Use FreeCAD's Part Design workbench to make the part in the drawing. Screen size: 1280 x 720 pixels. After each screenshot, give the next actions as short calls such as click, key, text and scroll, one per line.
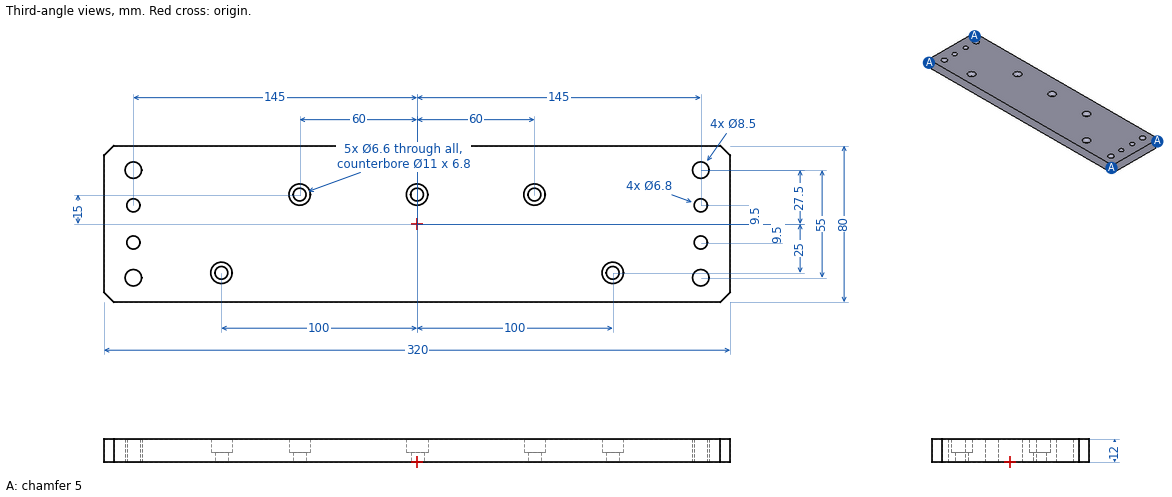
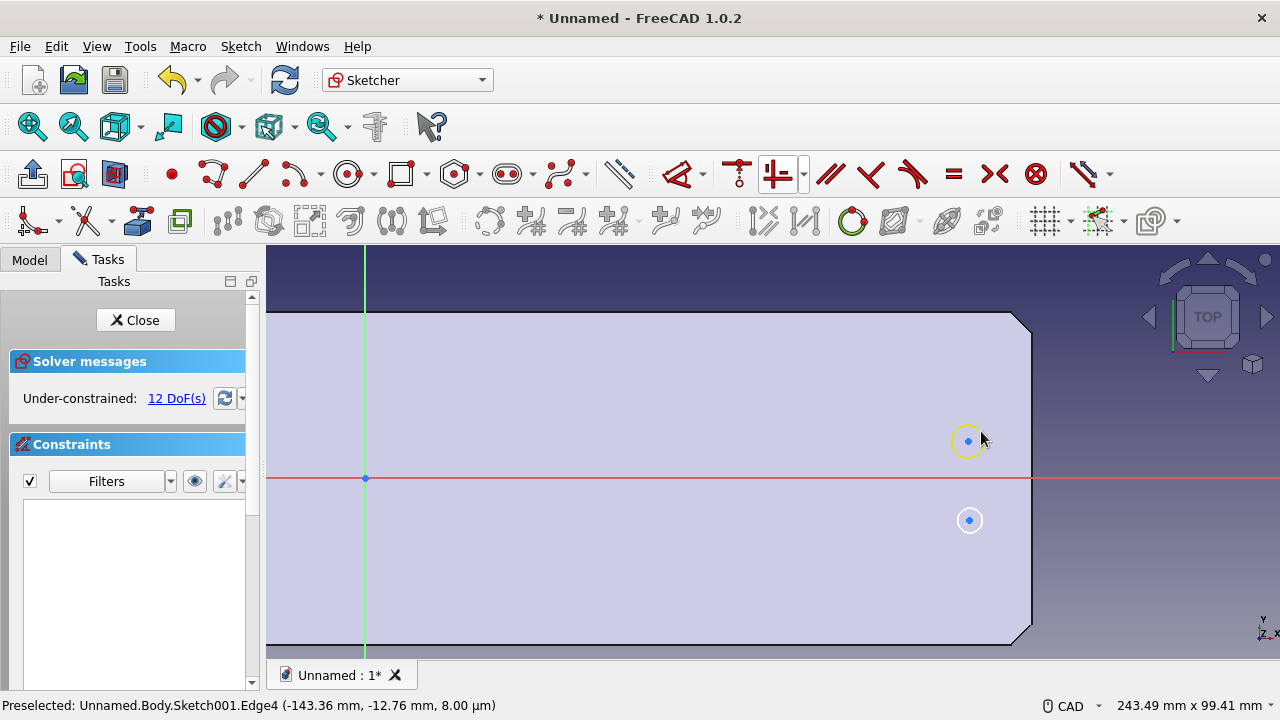
click(980, 430)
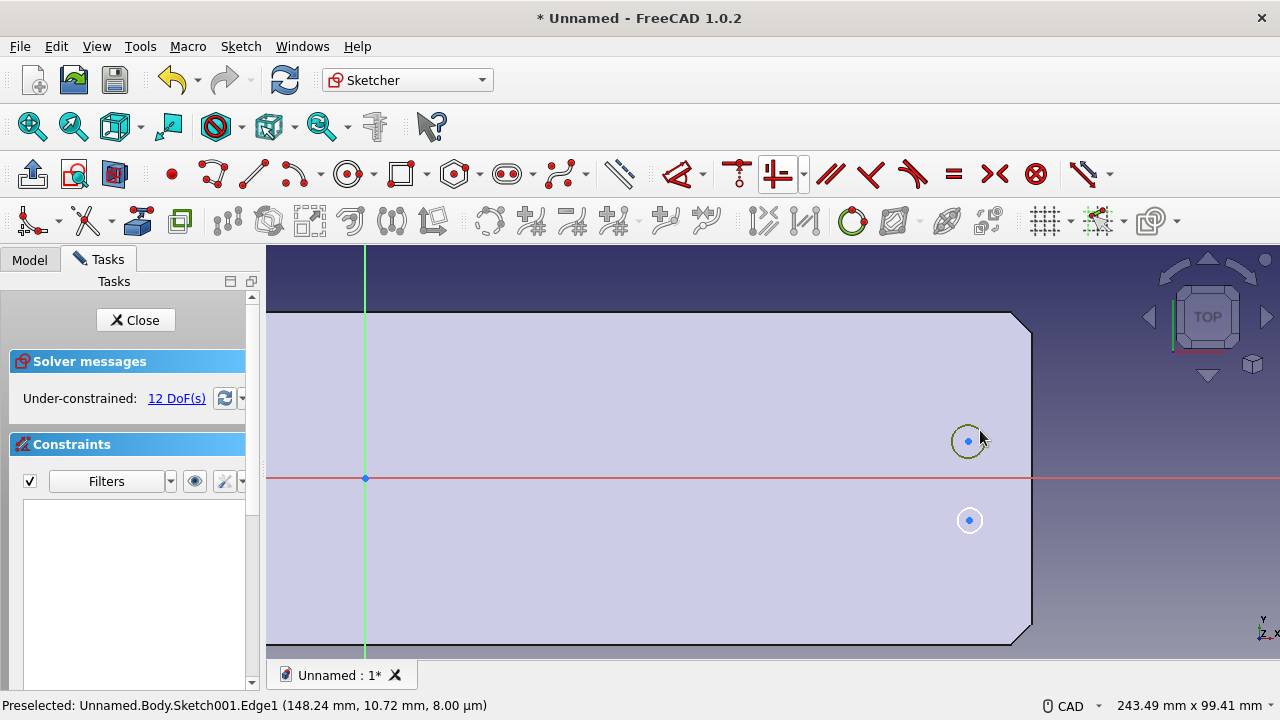
click(979, 512)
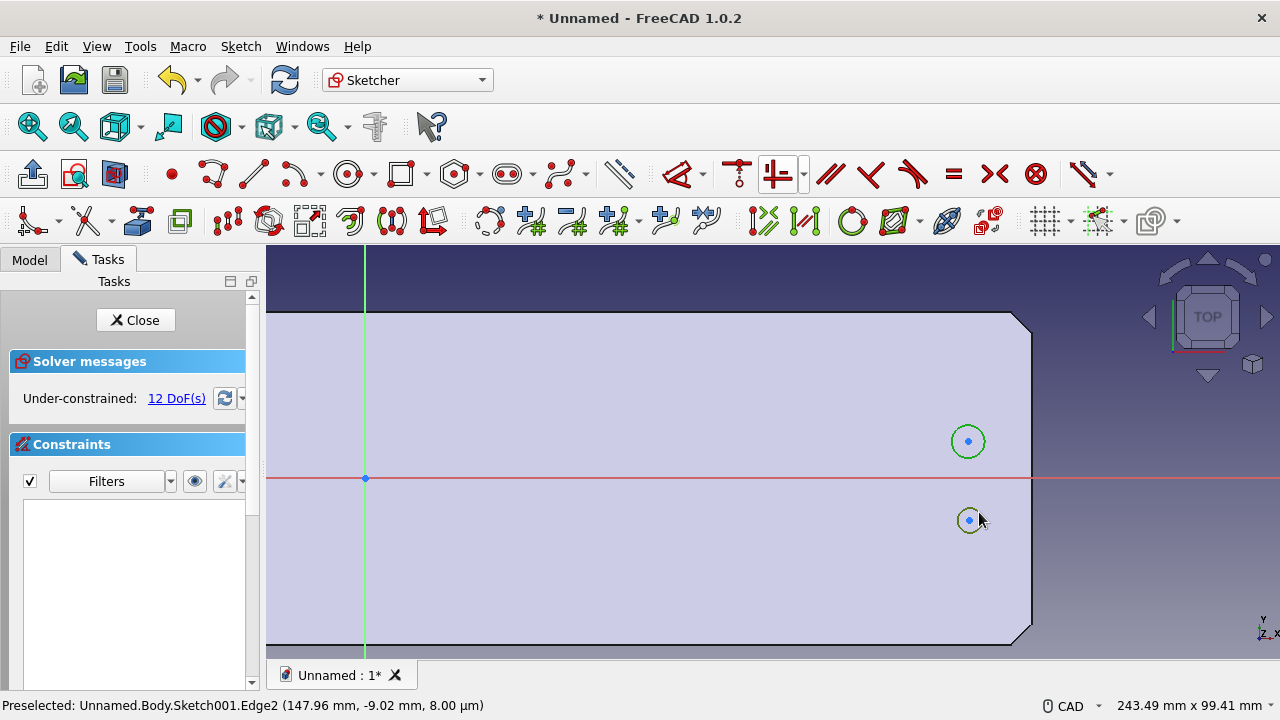
scroll(981, 430, down, 4)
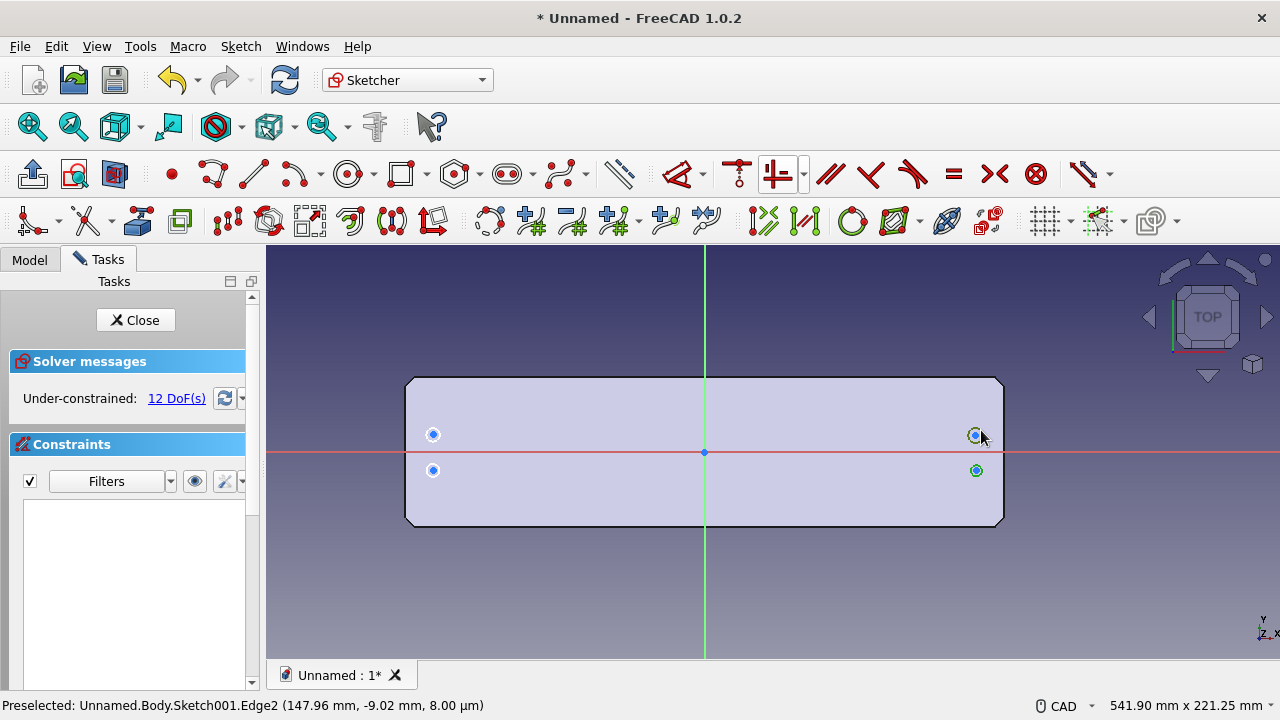
scroll(438, 430, up, 4)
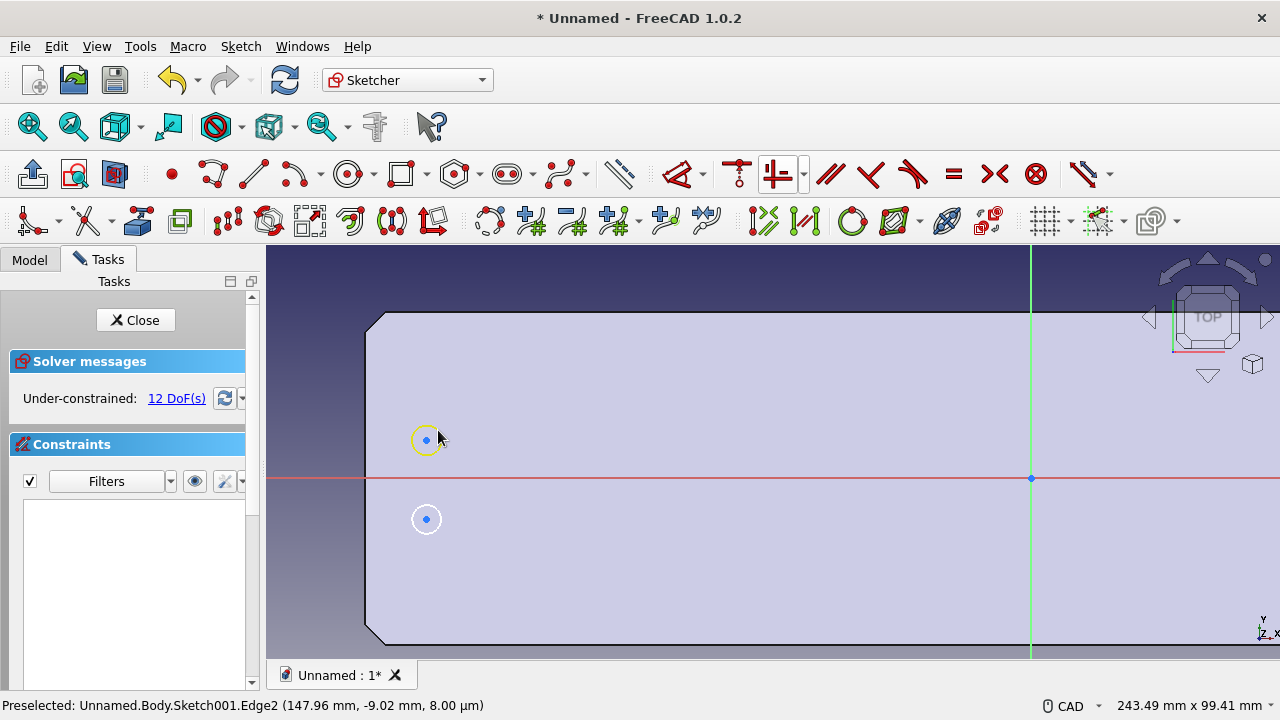
click(437, 430)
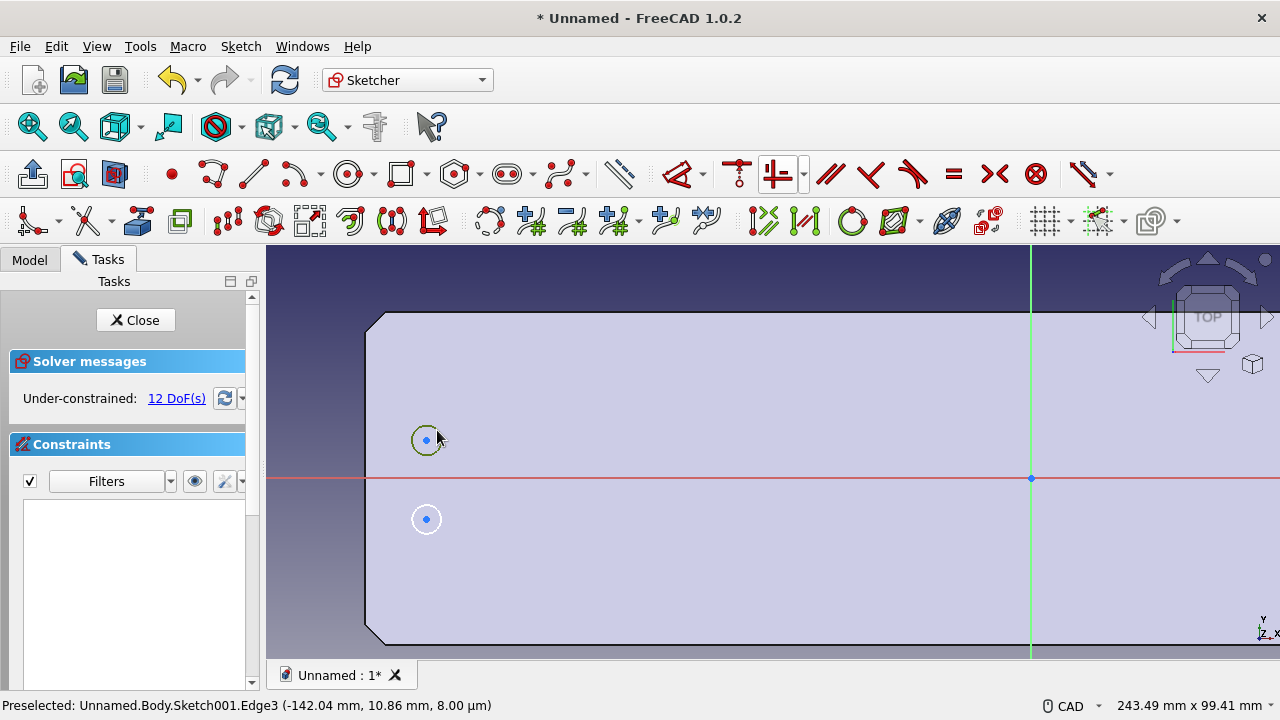
click(437, 509)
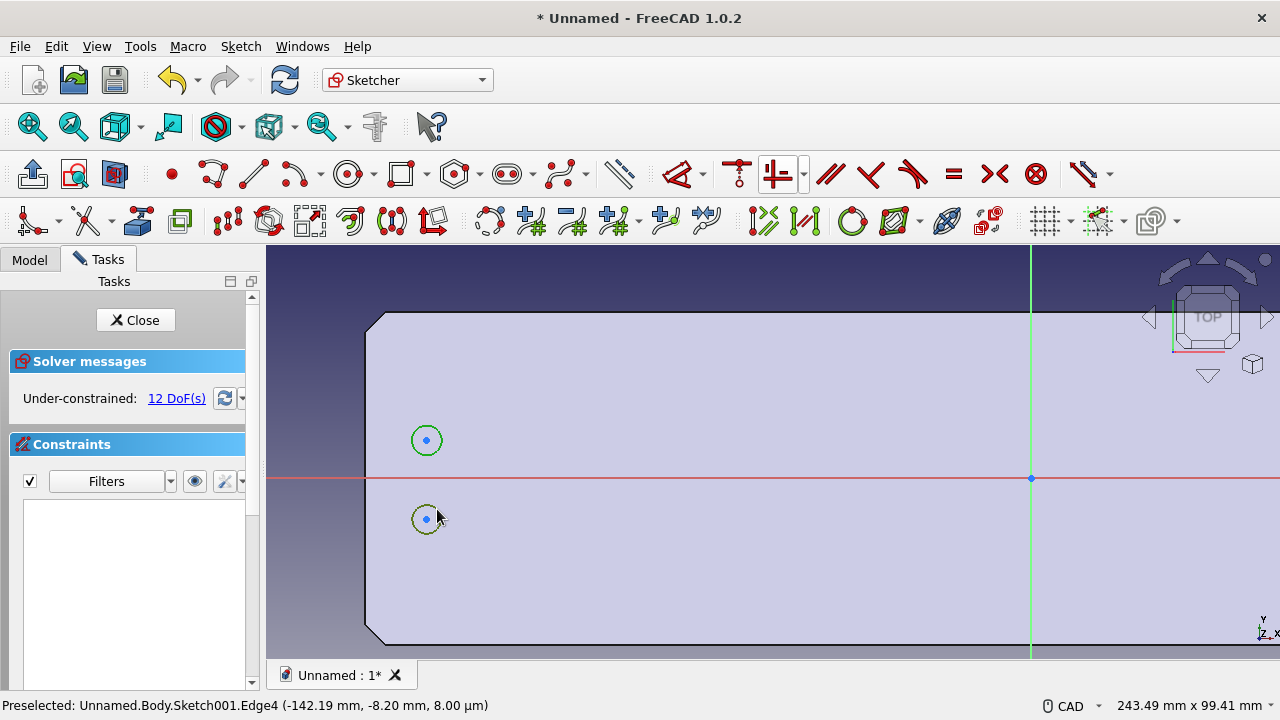
click(954, 174)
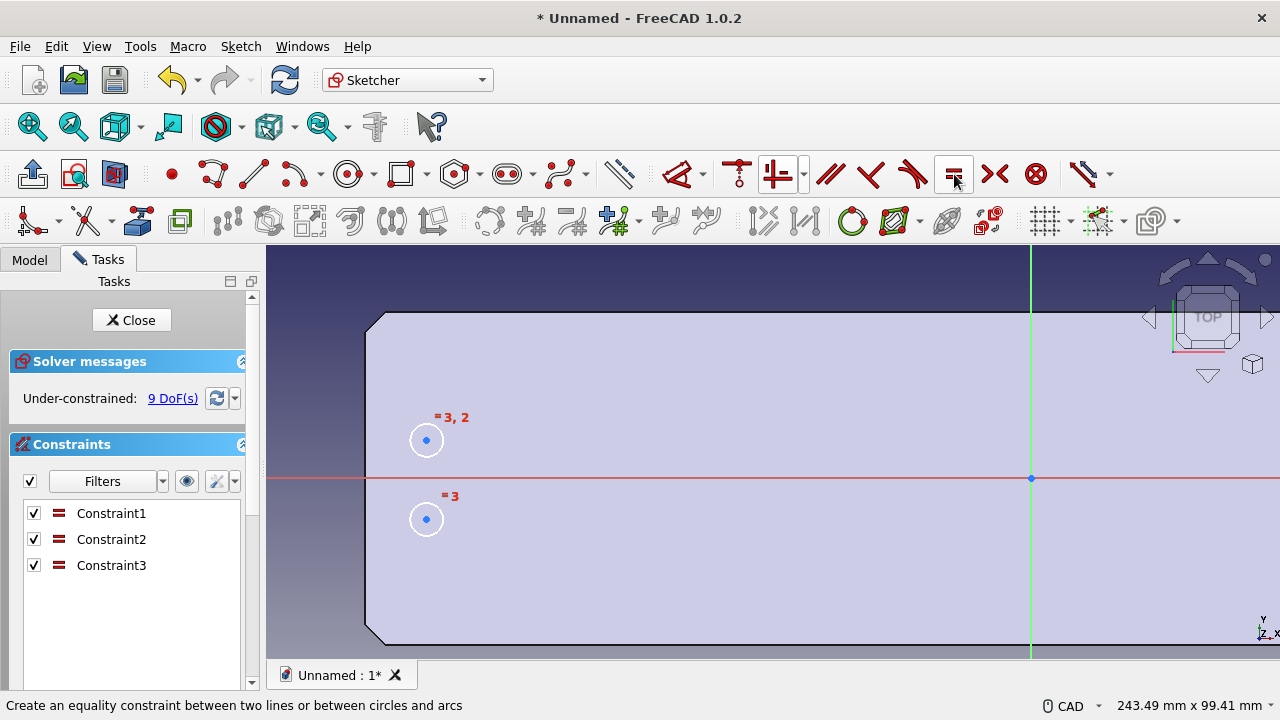
key(d)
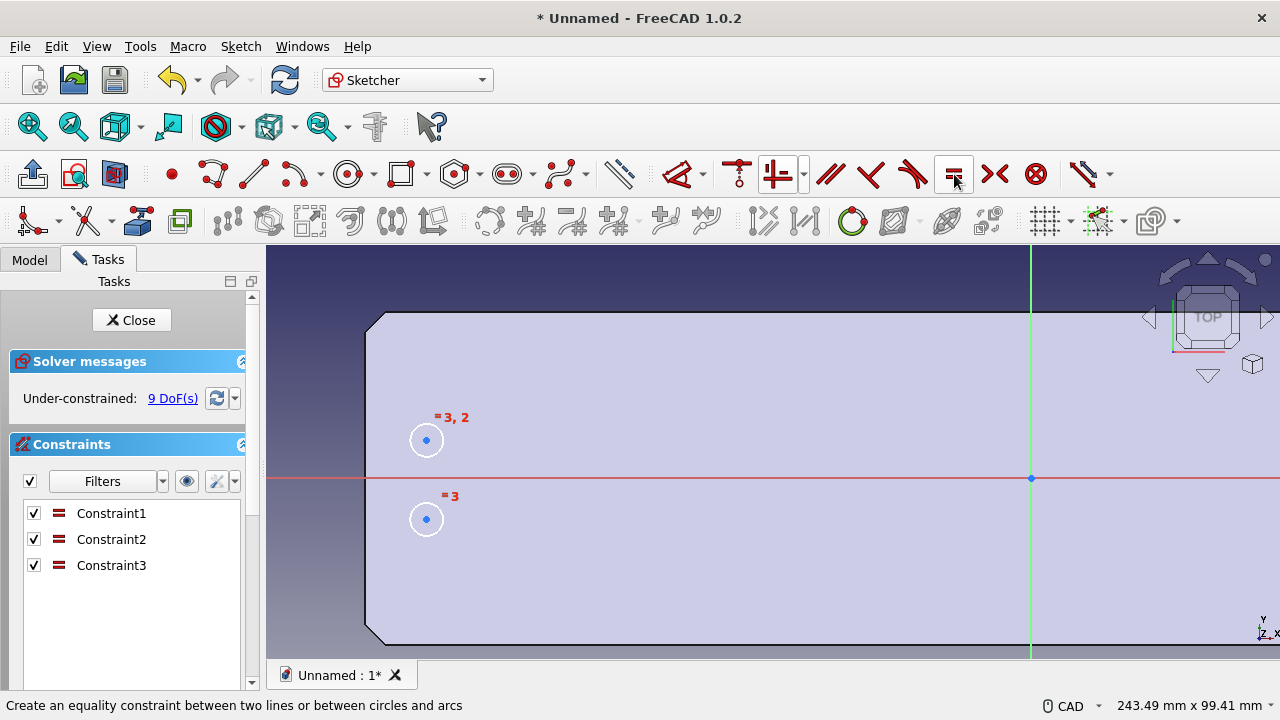
scroll(438, 430, down, 4)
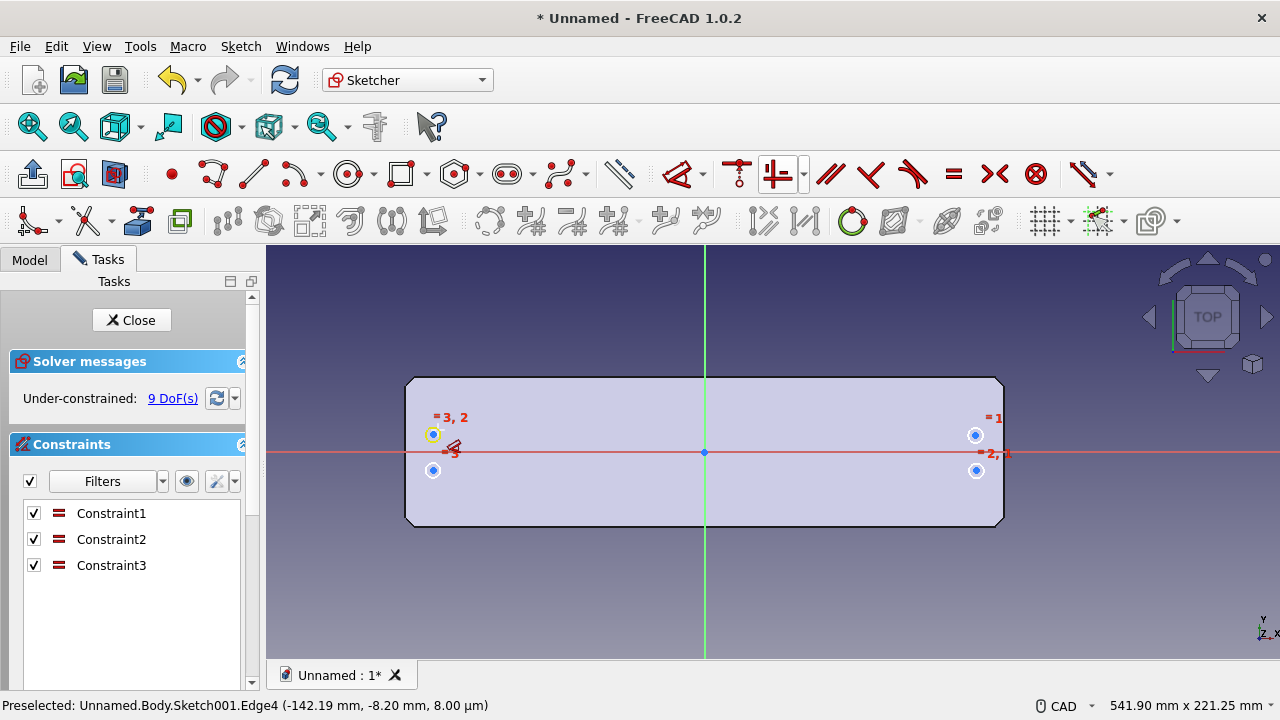
scroll(981, 430, up, 6)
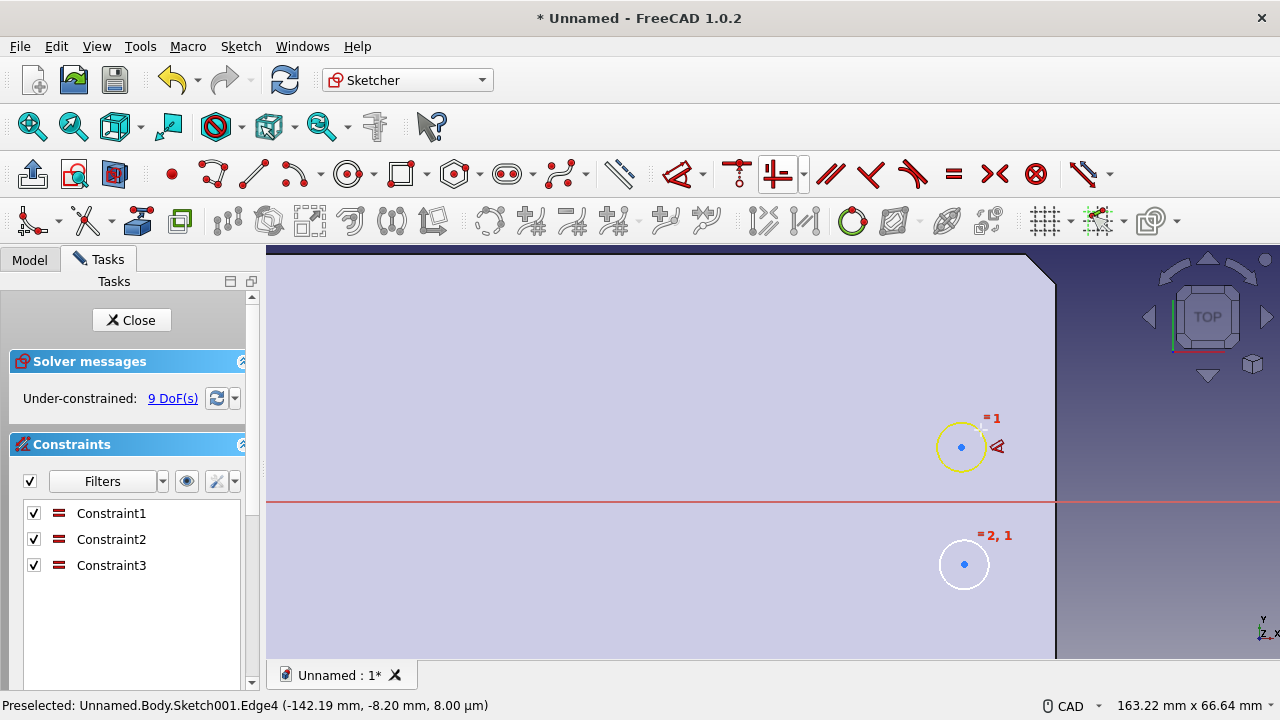
click(979, 430)
click(1002, 408)